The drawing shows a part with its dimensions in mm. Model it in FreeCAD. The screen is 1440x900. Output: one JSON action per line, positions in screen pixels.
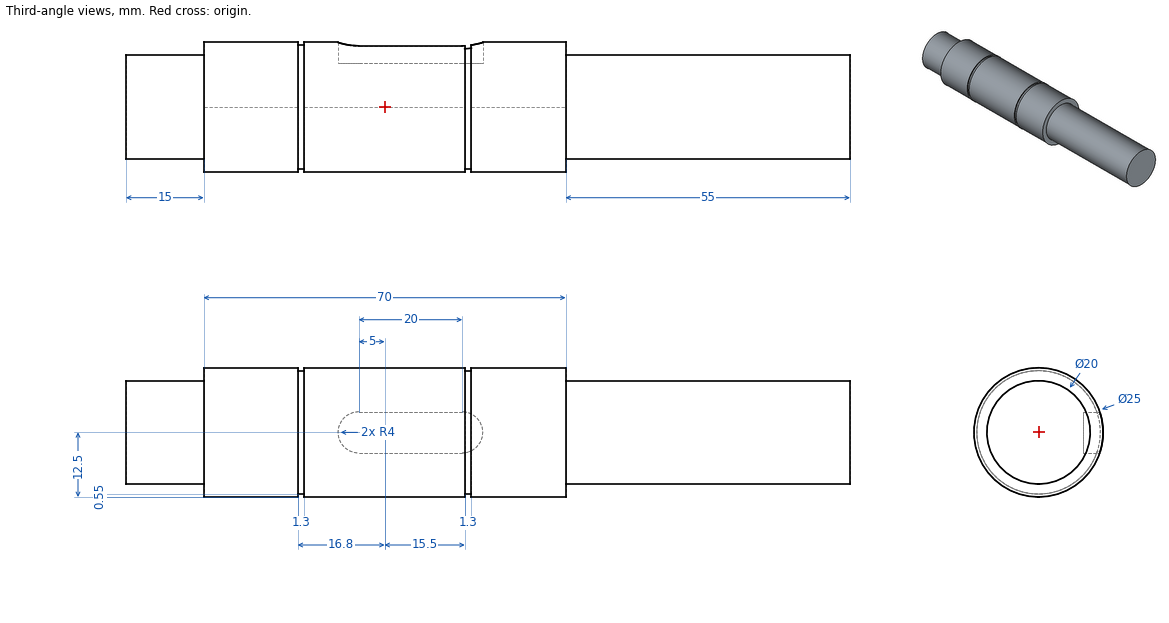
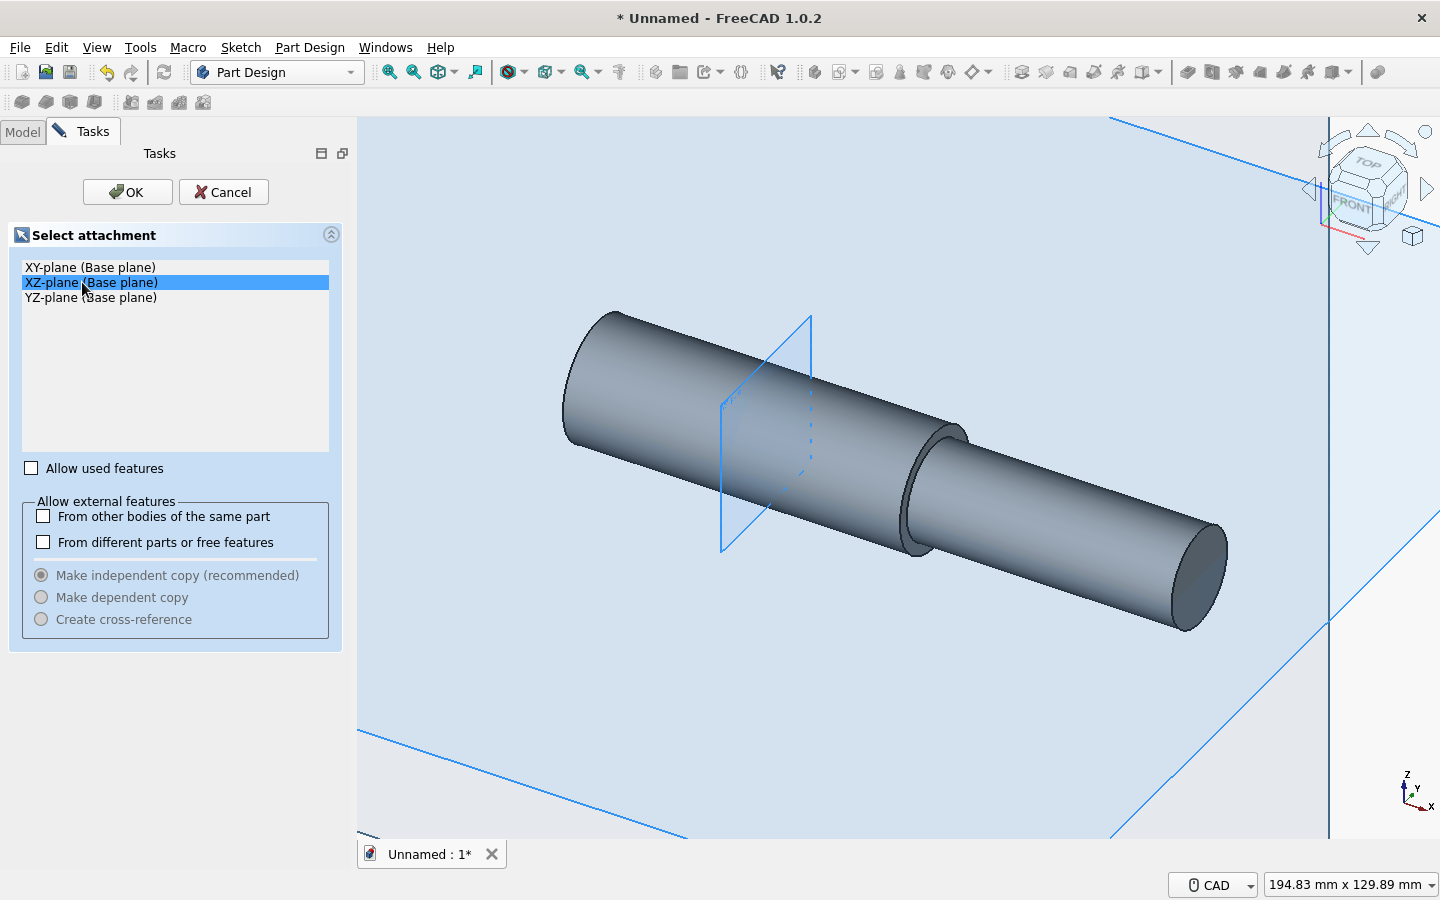
{"action": "left_click", "coordinate": [128, 192]}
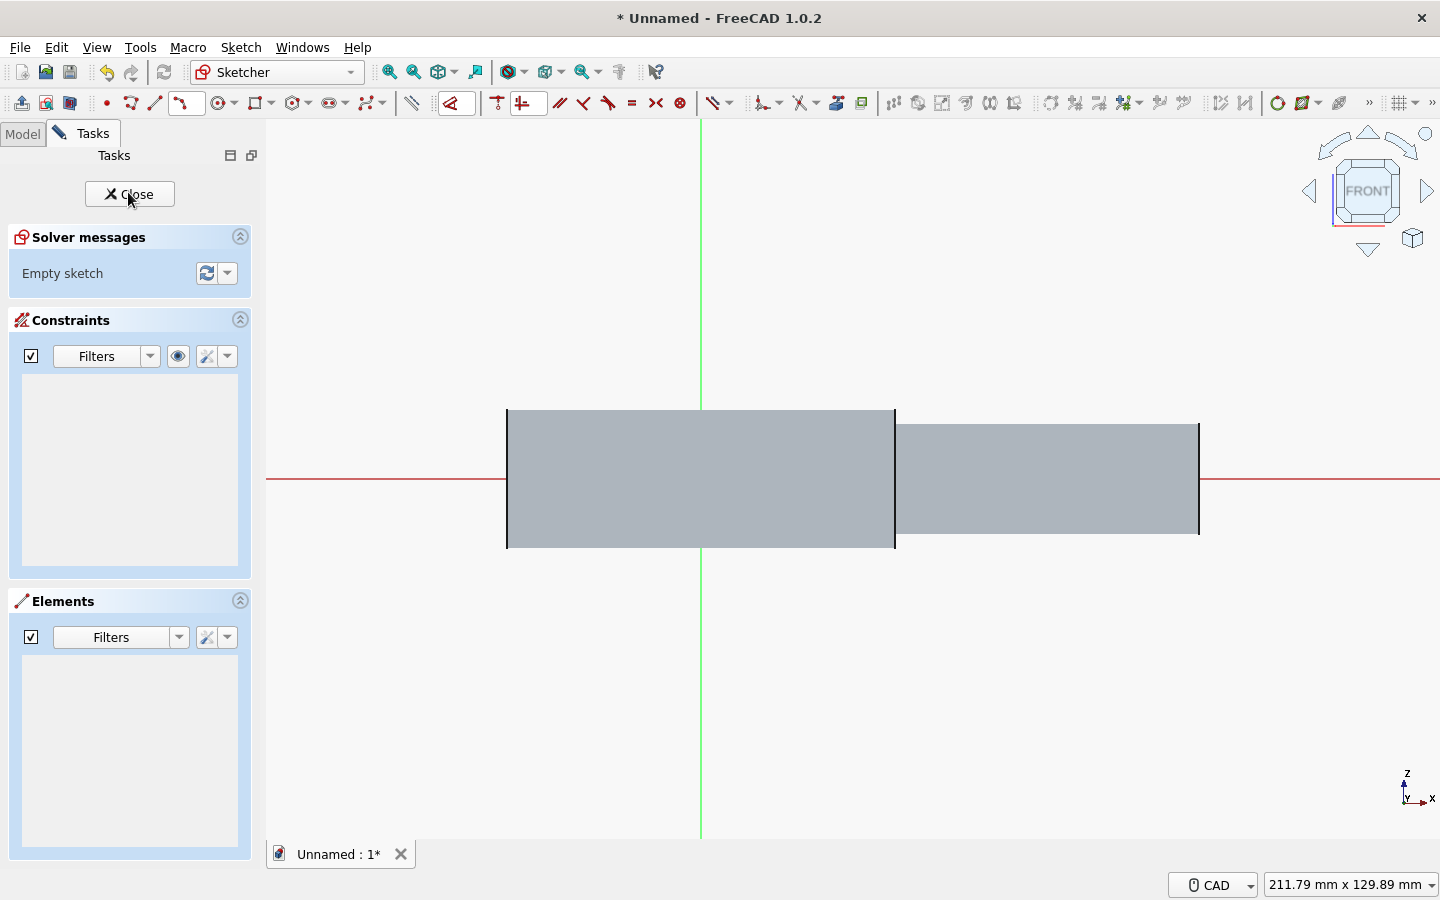
{"action": "key", "text": "q s"}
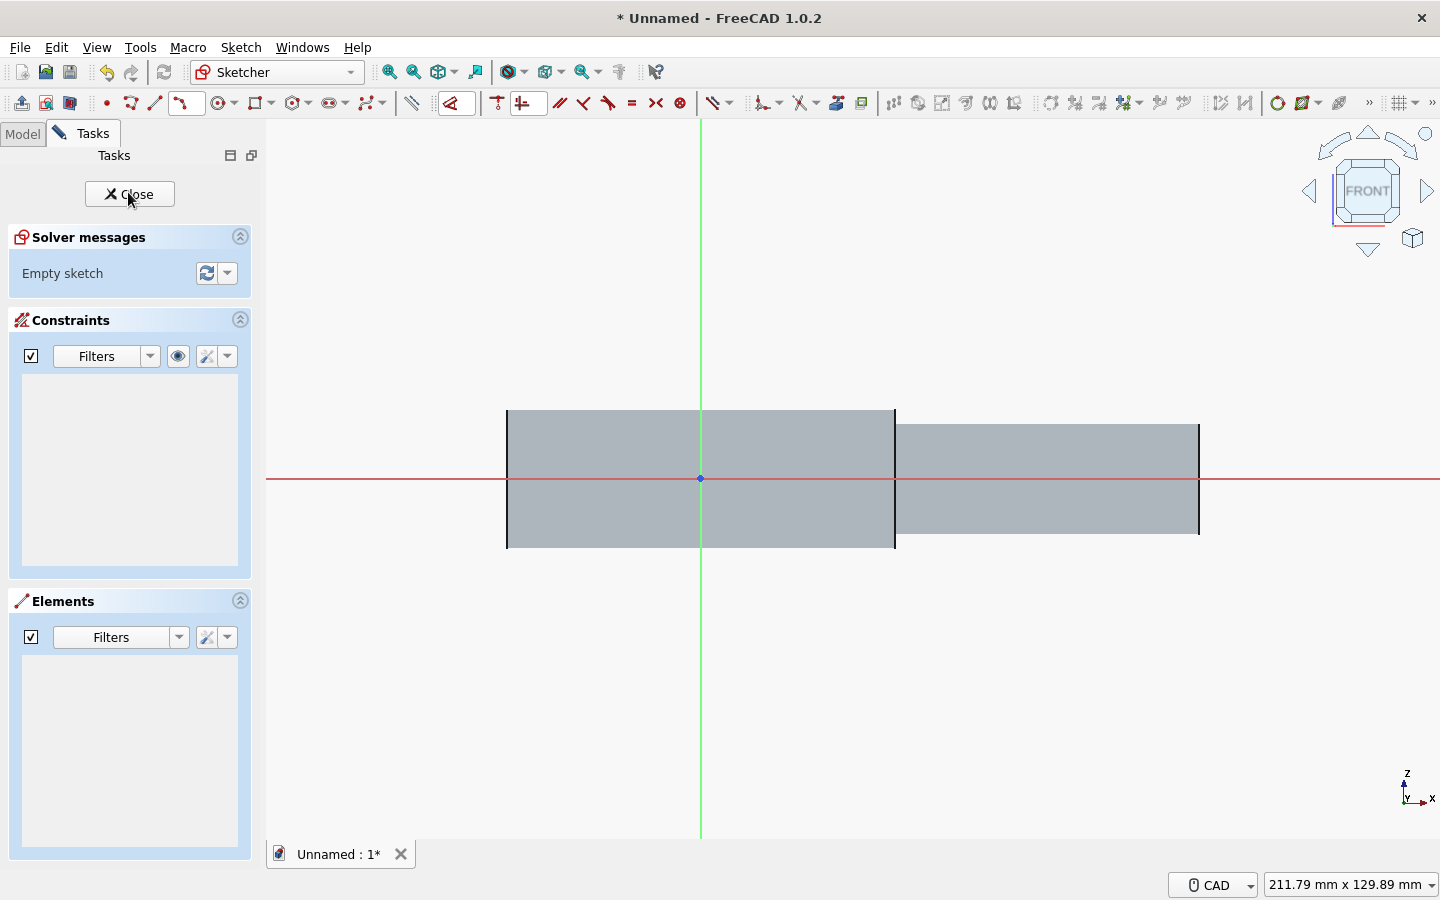
{"action": "scroll", "coordinate": [673, 525], "scroll_direction": "up", "scroll_amount": 7}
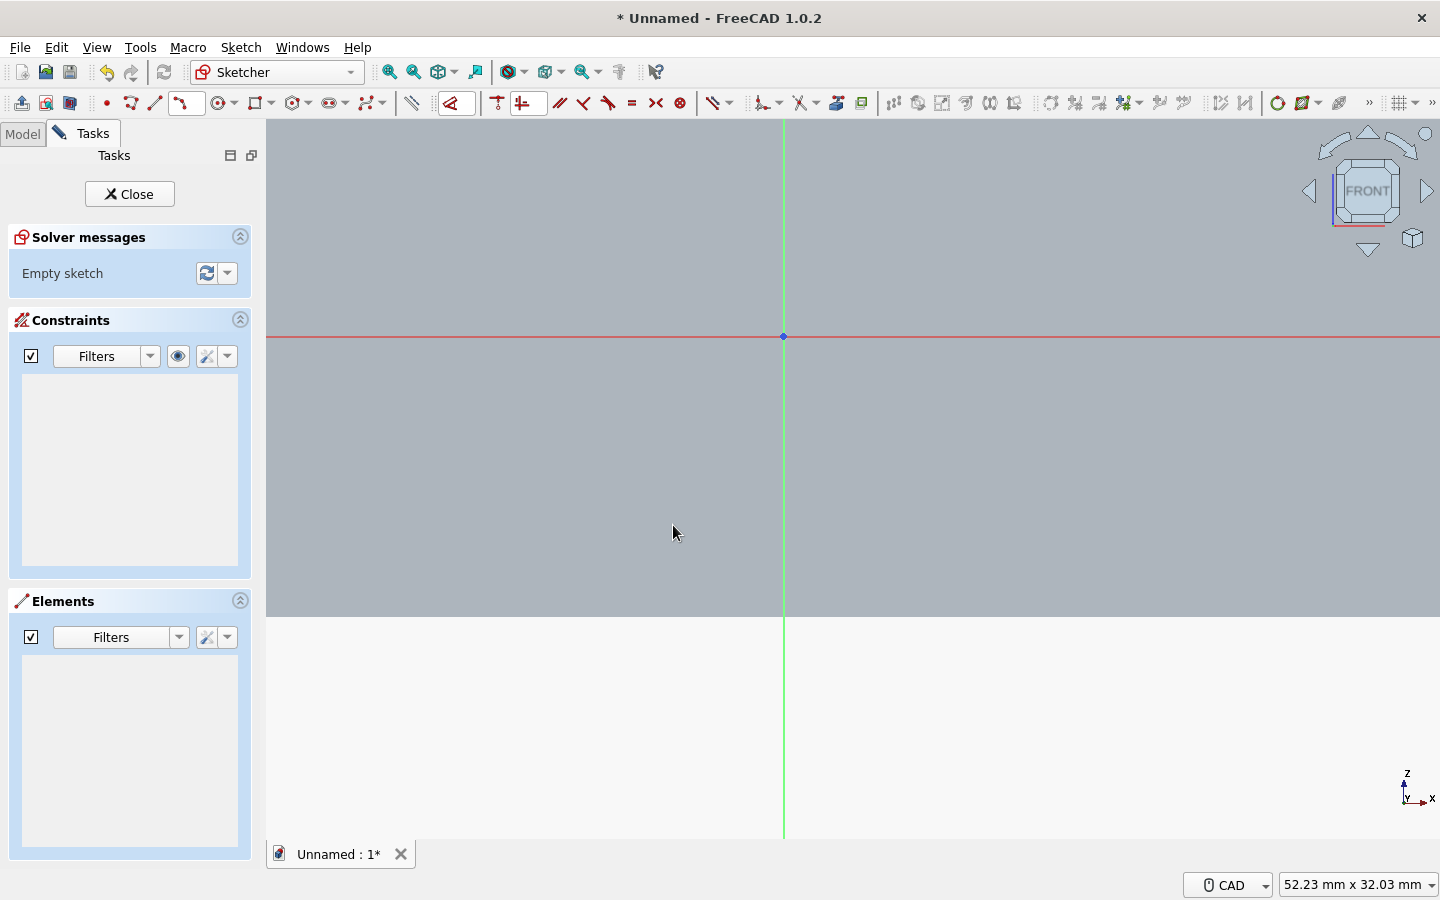
{"action": "left_click", "coordinate": [256, 104]}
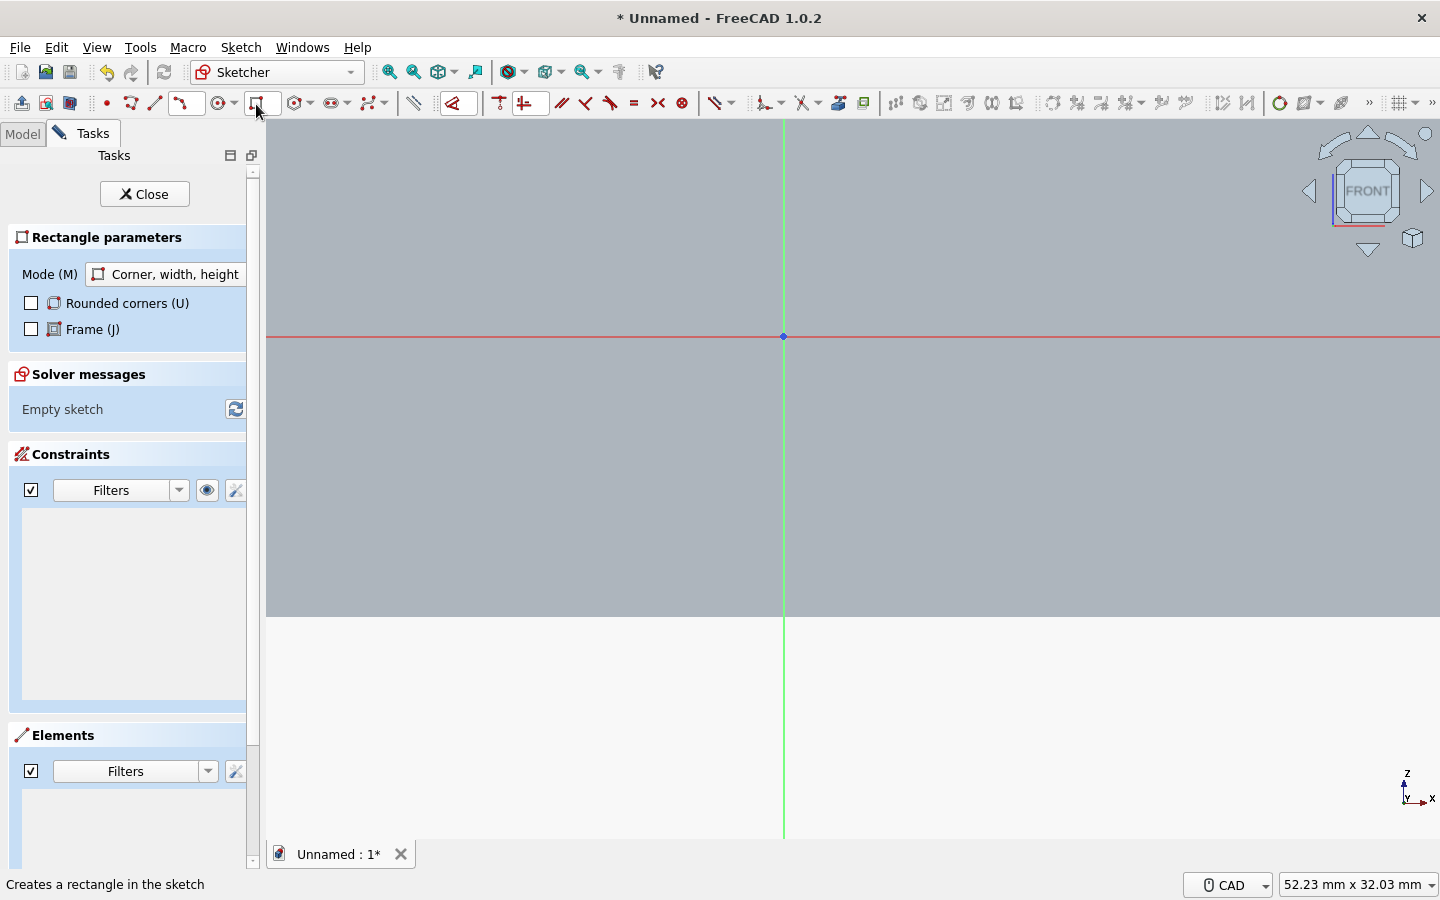
{"action": "scroll", "coordinate": [406, 605], "scroll_direction": "up", "scroll_amount": 2}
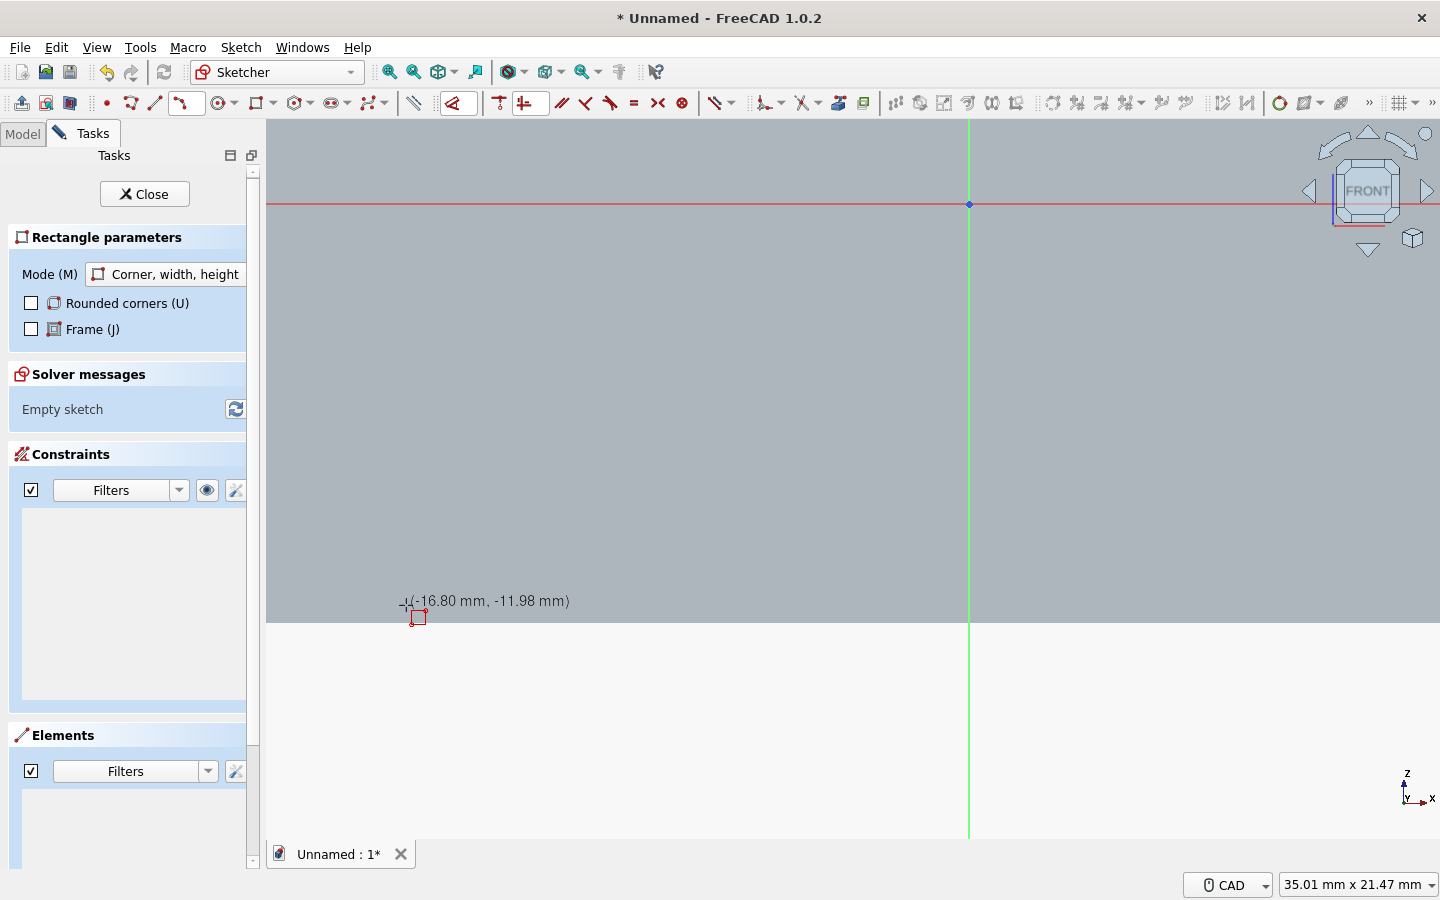
{"action": "left_click", "coordinate": [406, 605]}
{"action": "left_click", "coordinate": [450, 624]}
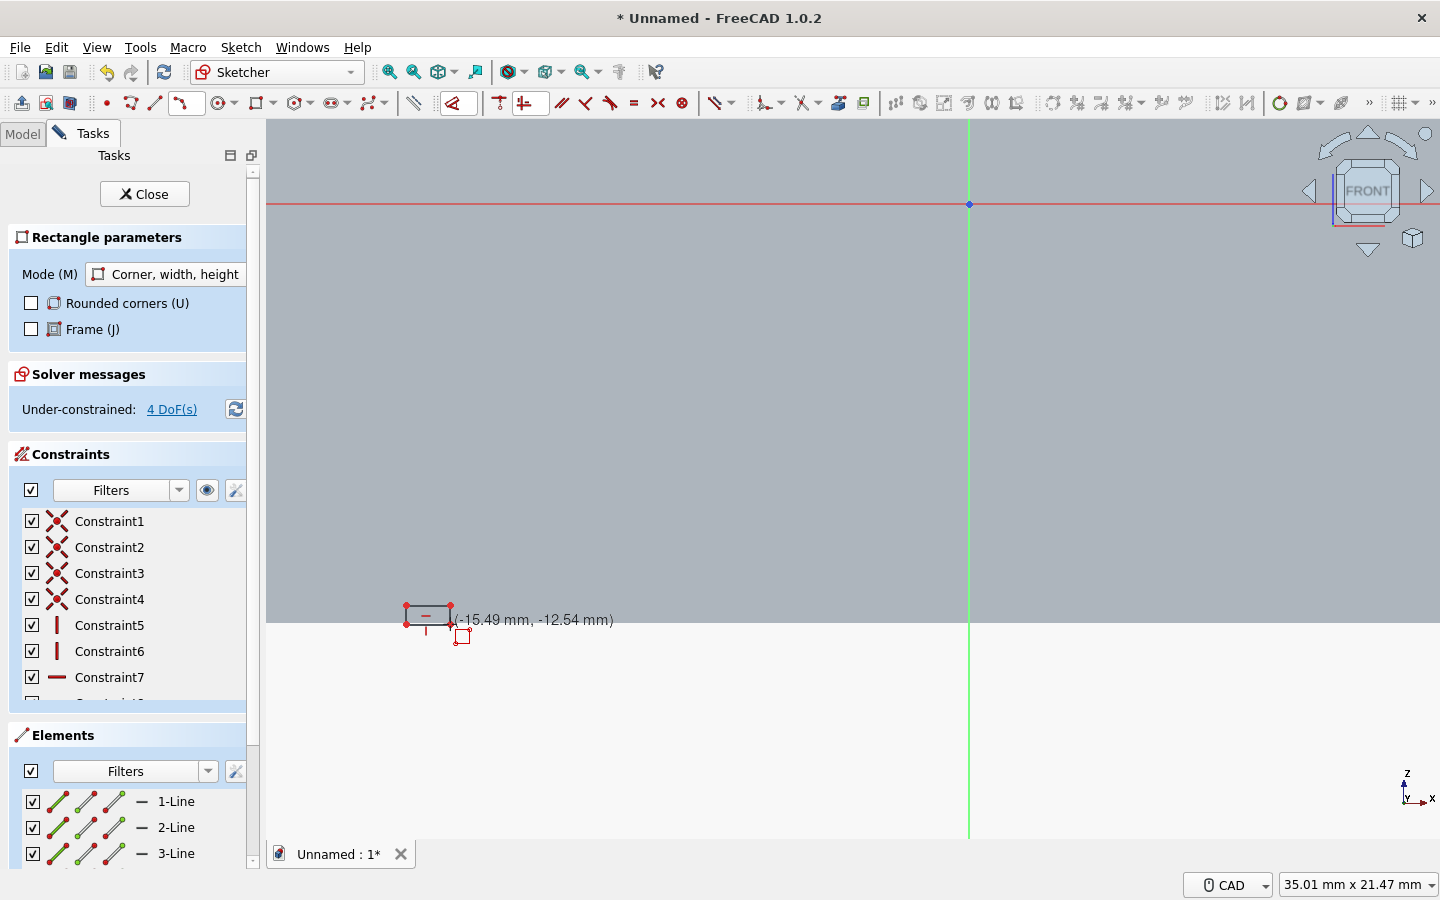
{"action": "scroll", "coordinate": [409, 611], "scroll_direction": "down", "scroll_amount": 2}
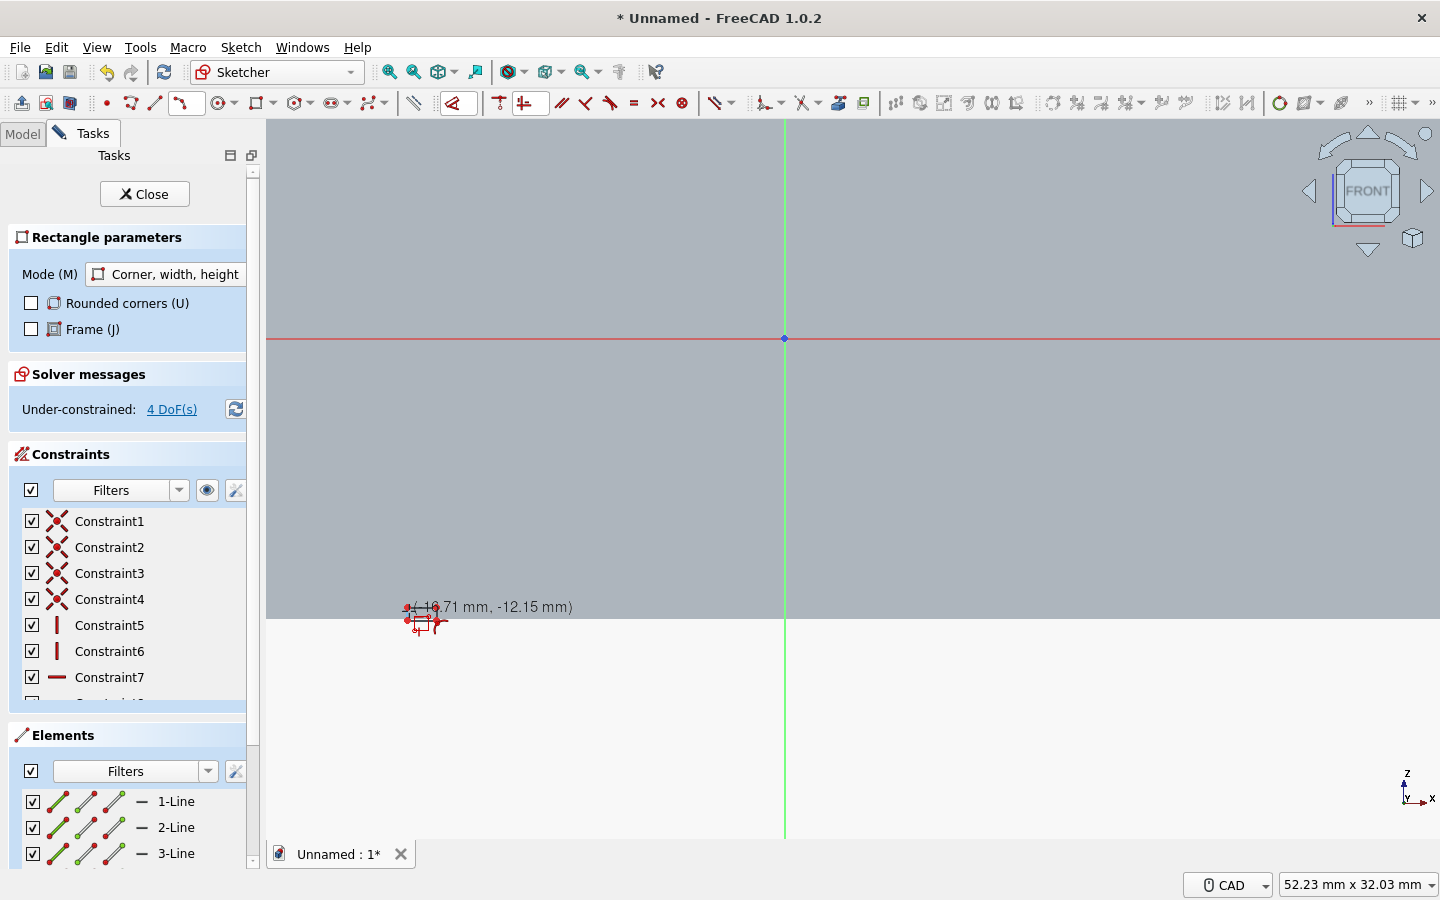
{"action": "scroll", "coordinate": [1133, 607], "scroll_direction": "up", "scroll_amount": 2}